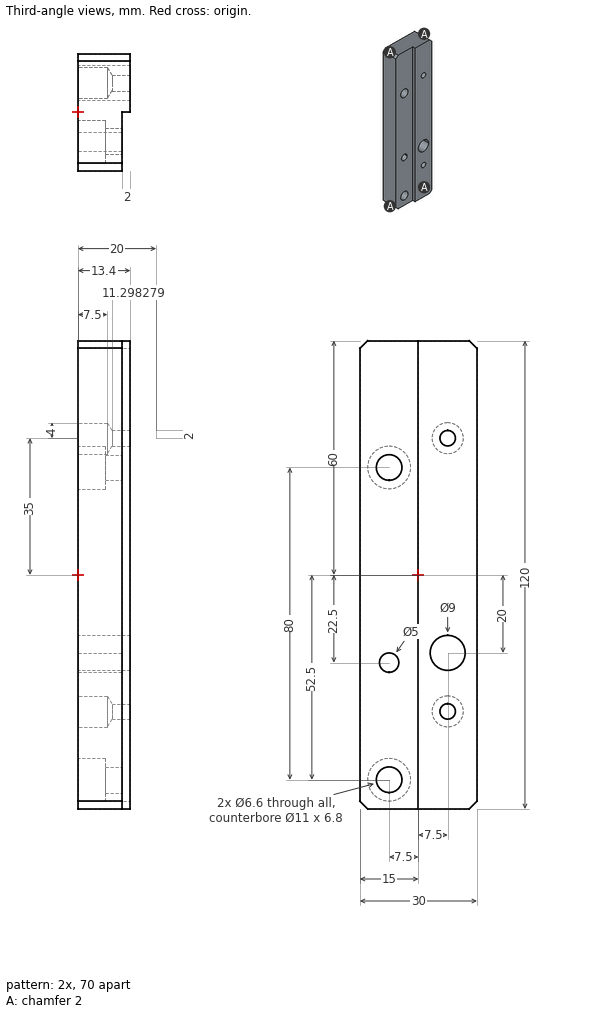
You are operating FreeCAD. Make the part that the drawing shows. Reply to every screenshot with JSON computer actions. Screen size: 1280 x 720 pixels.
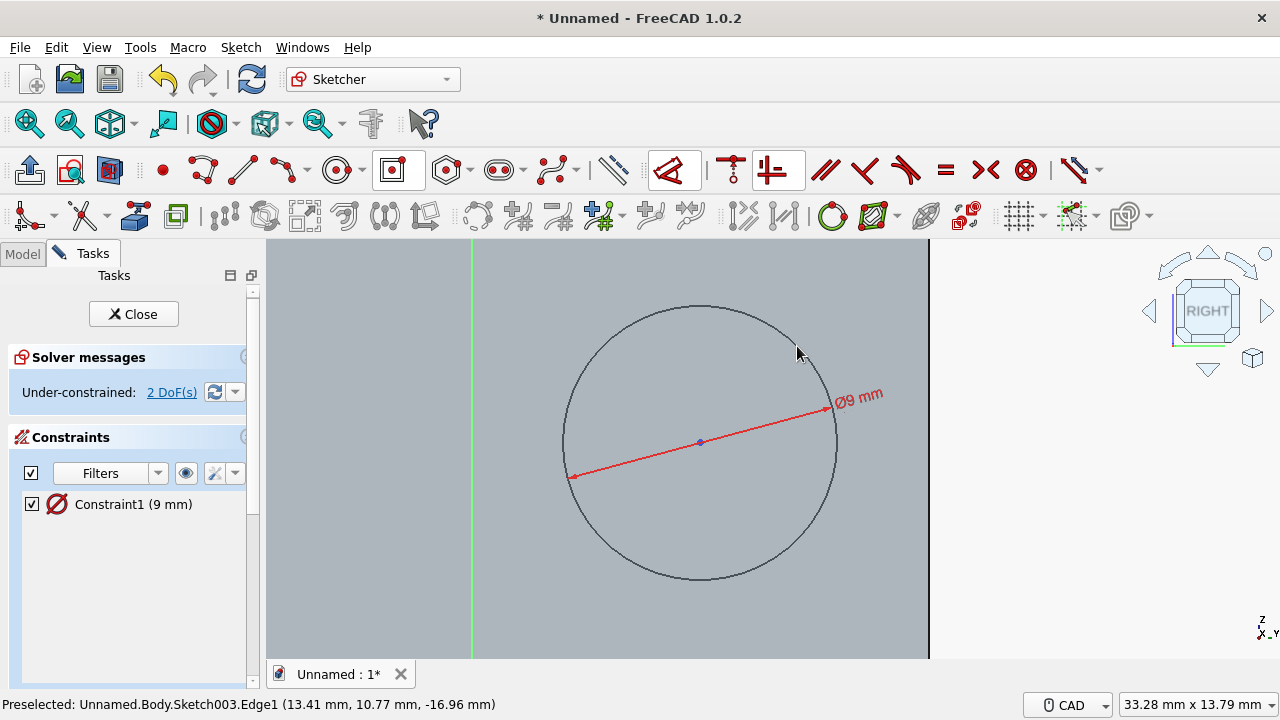
{"action": "left_click", "coordinate": [700, 443]}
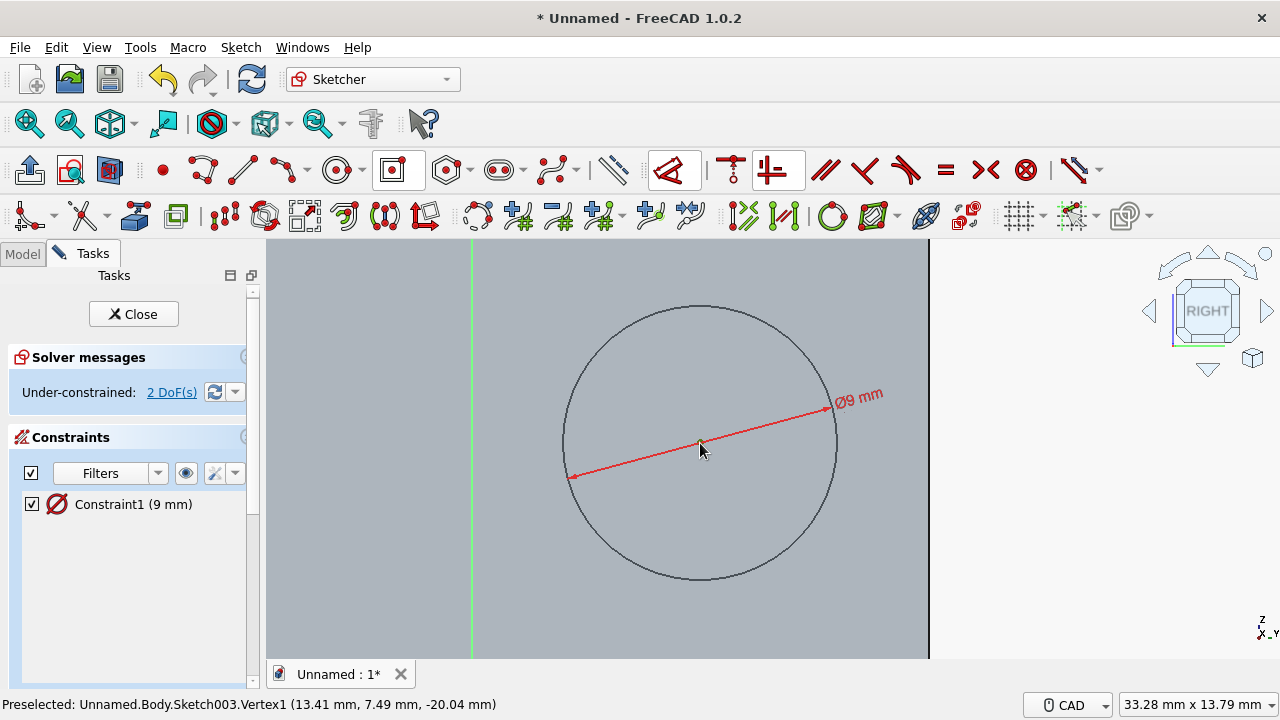
{"action": "left_click", "coordinate": [696, 170]}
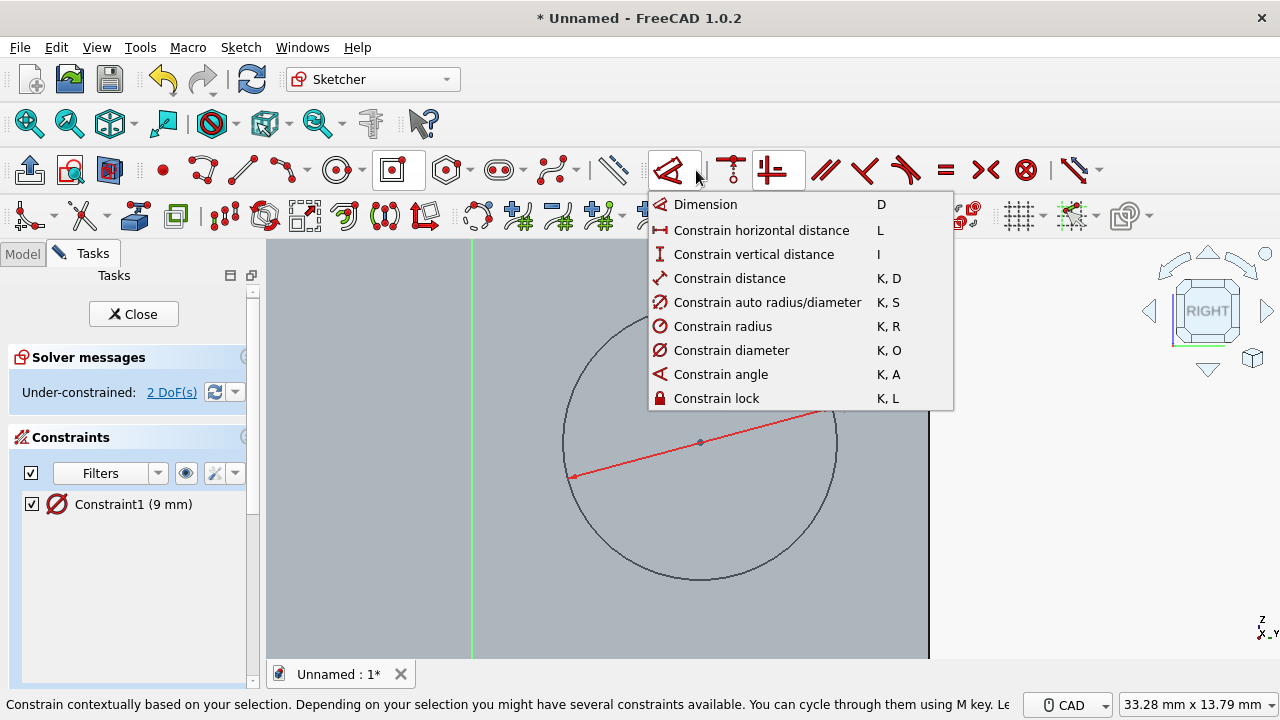
{"action": "left_click", "coordinate": [801, 254]}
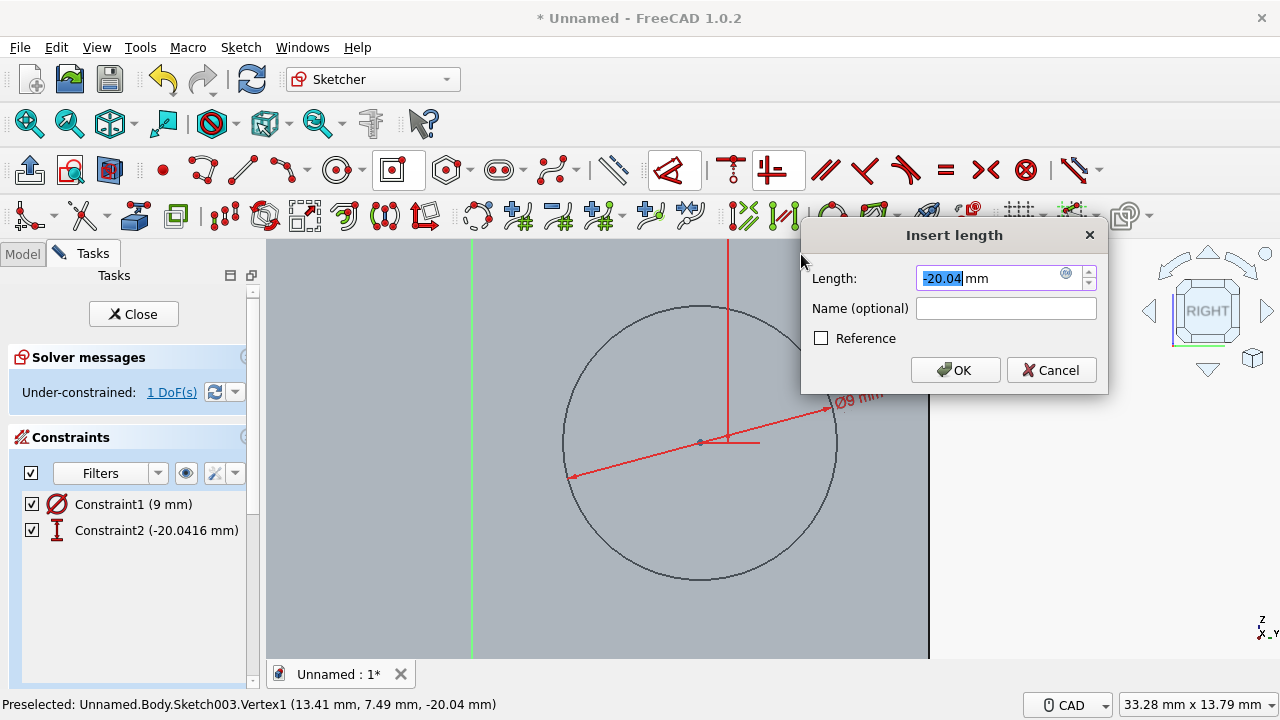
{"action": "type", "text": "-20"}
{"action": "key", "text": "Return"}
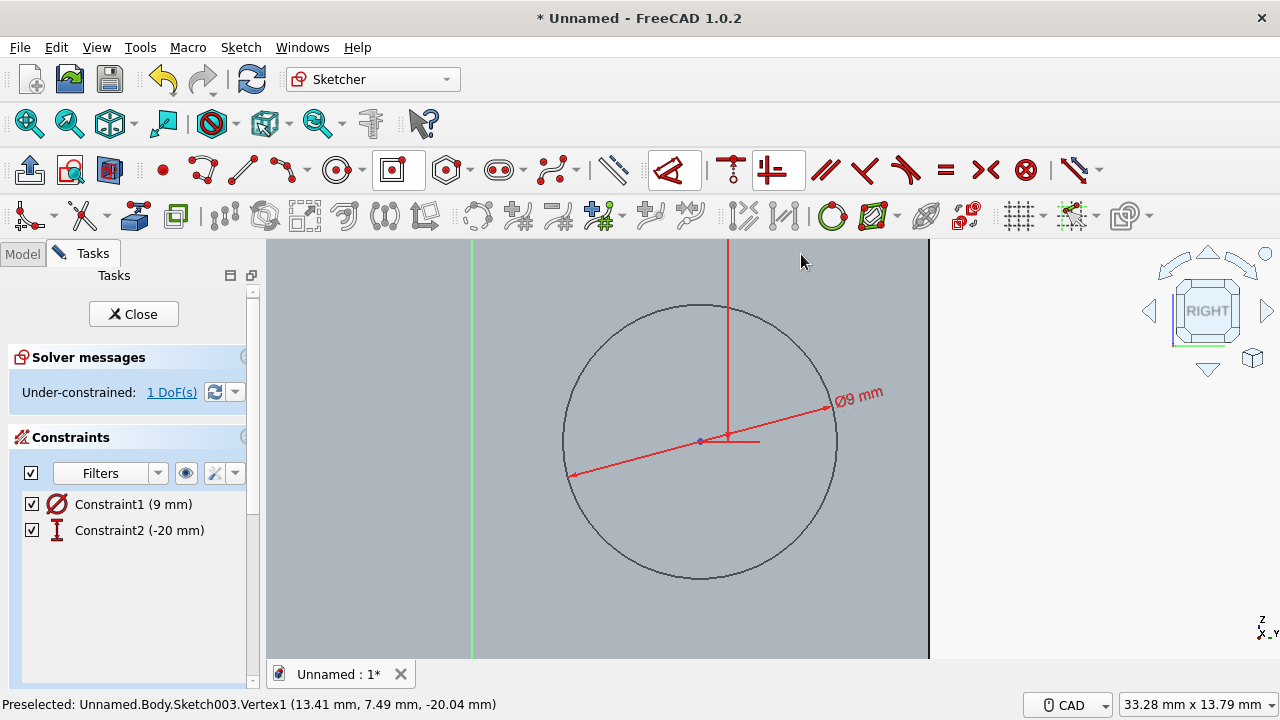
{"action": "left_click", "coordinate": [700, 442]}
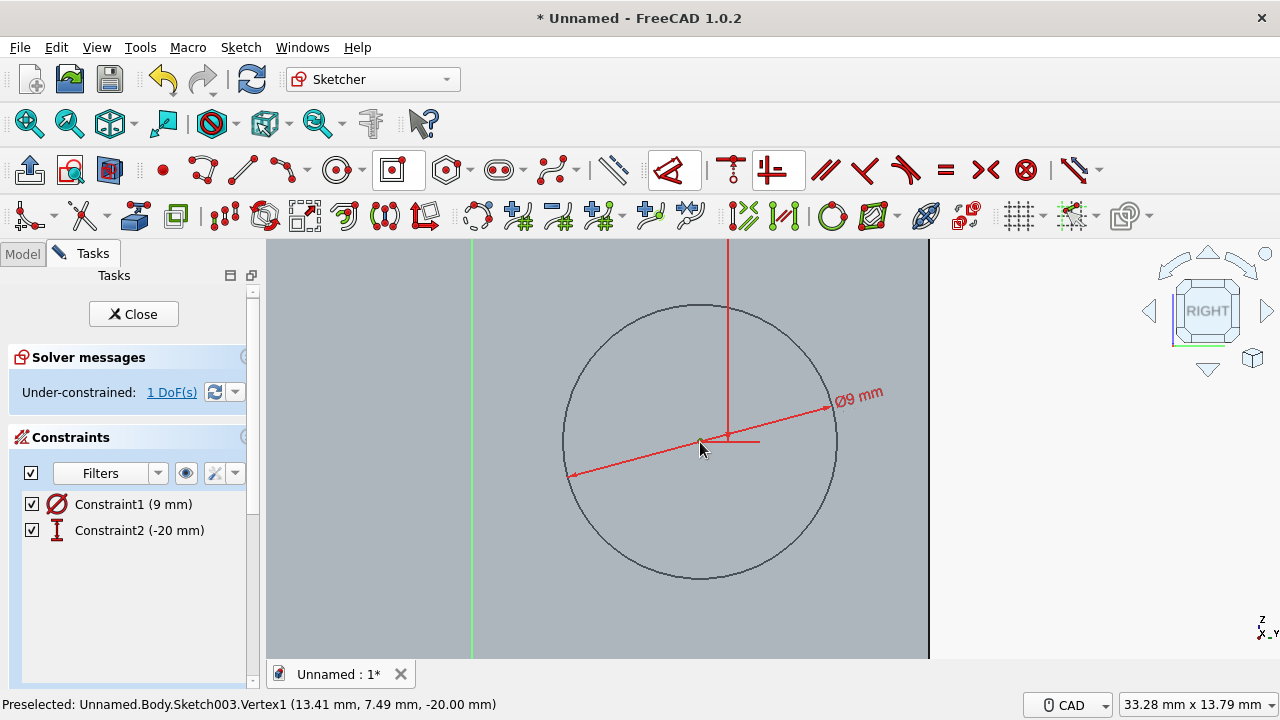
{"action": "key", "text": "l"}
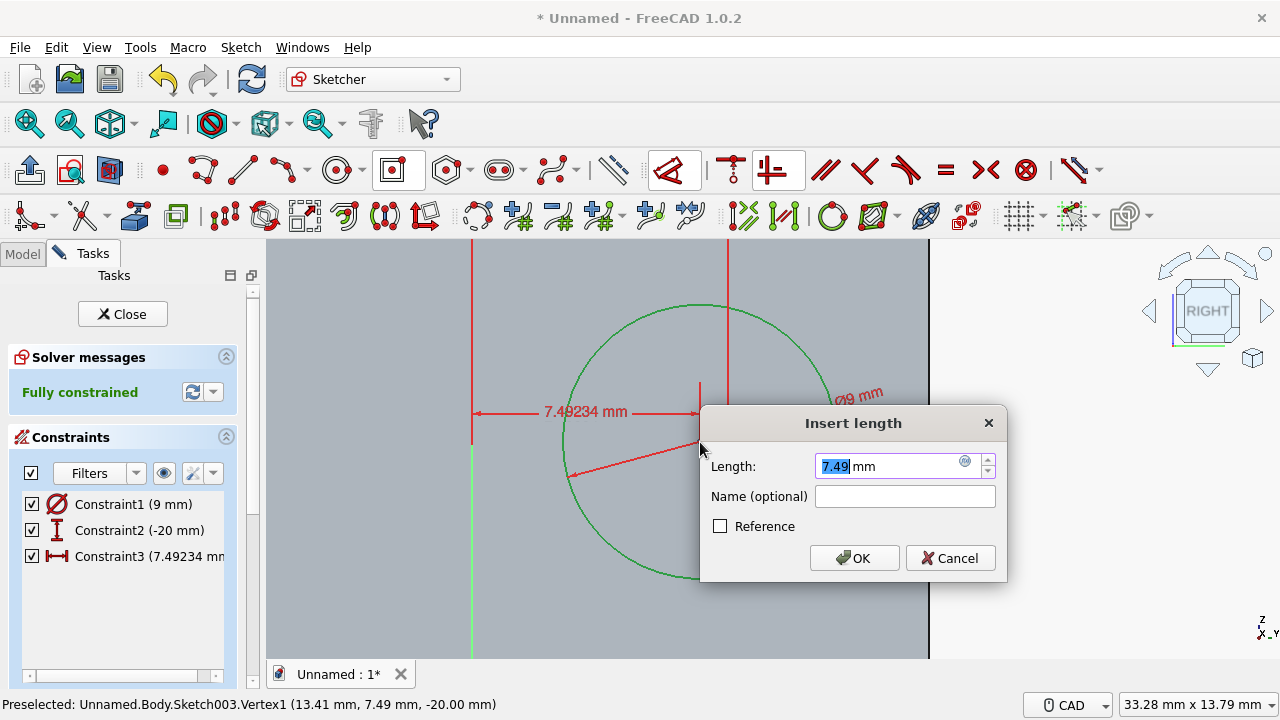
{"action": "type", "text": "7.5"}
{"action": "key", "text": "Return"}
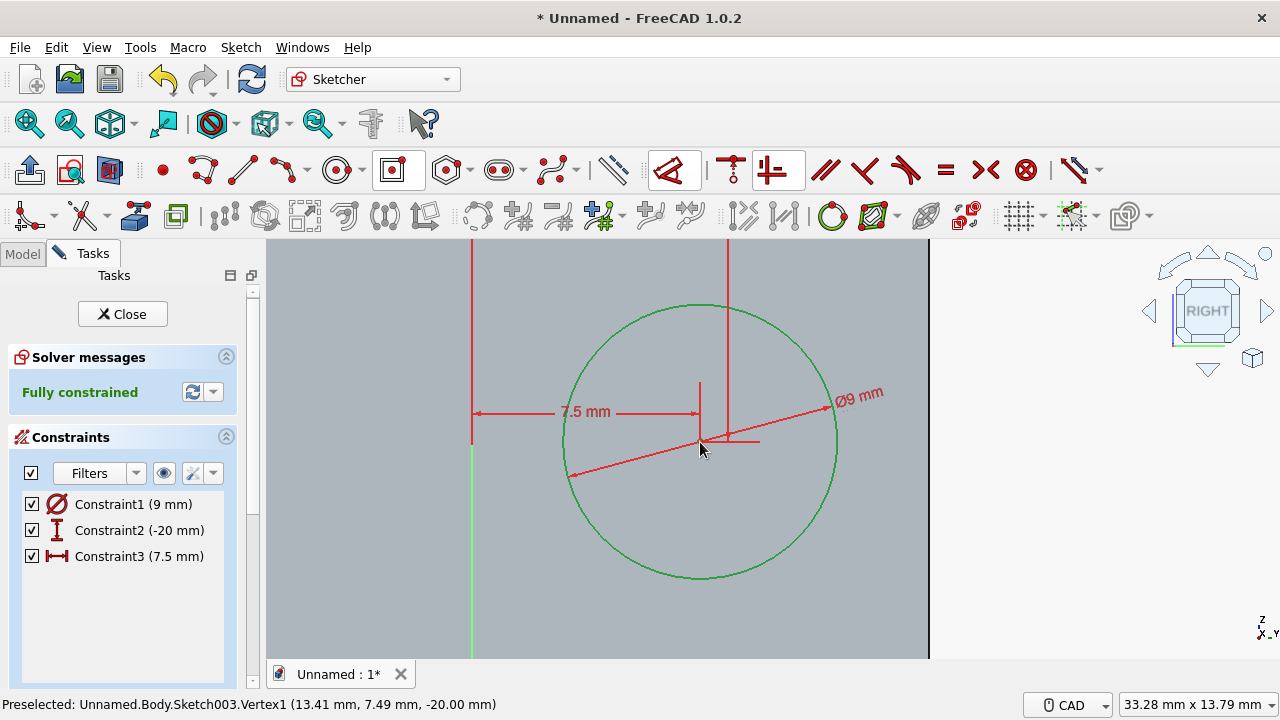
{"action": "left_click", "coordinate": [123, 314]}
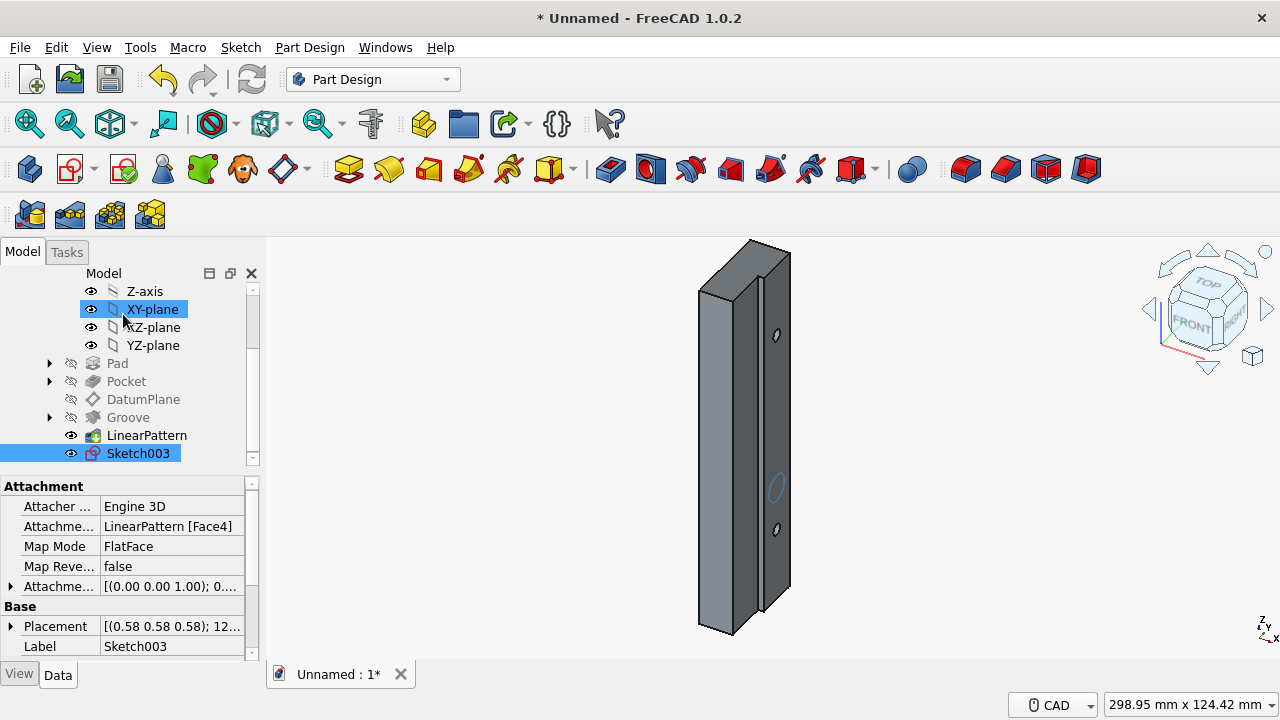
{"action": "left_click", "coordinate": [612, 170]}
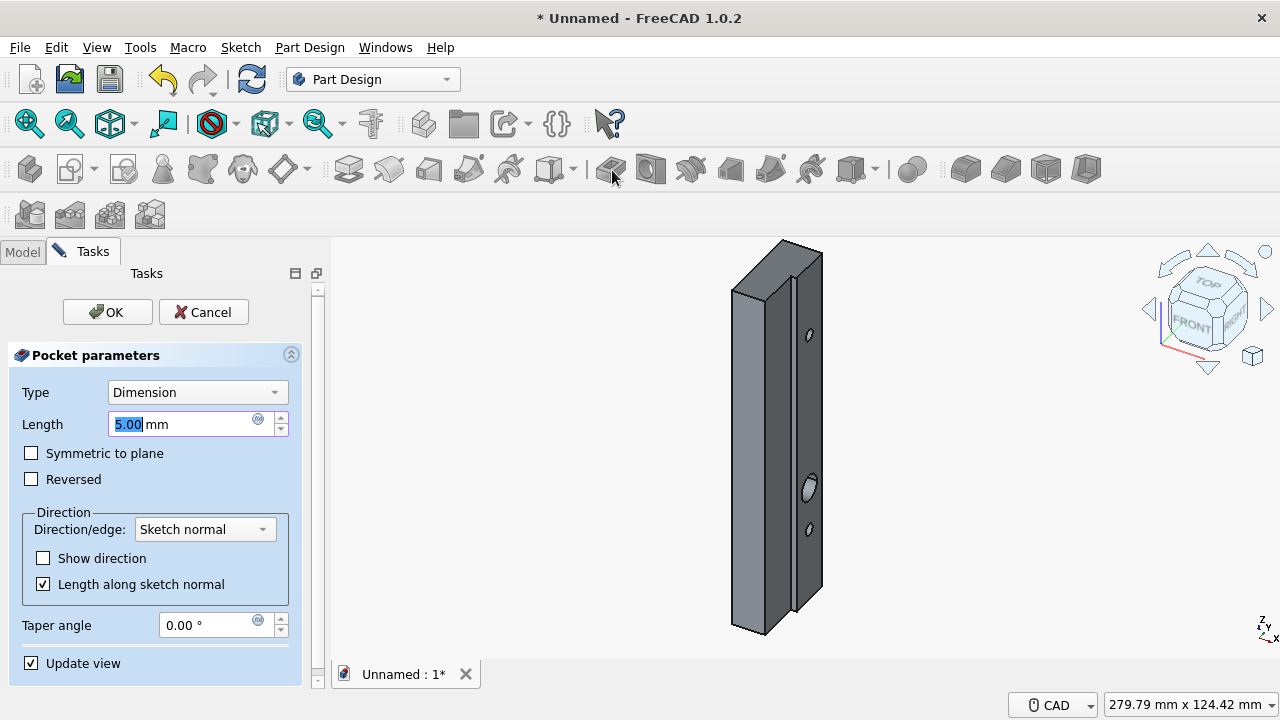
{"action": "left_click", "coordinate": [198, 392]}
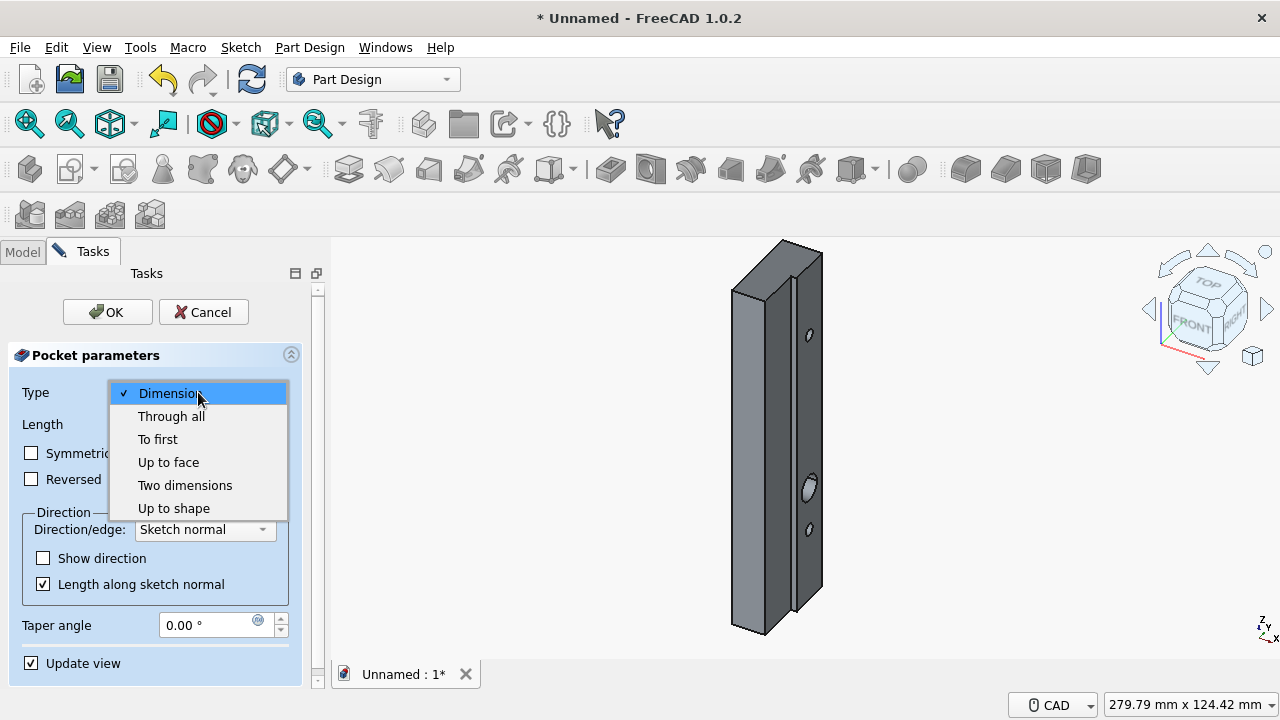
{"action": "left_click", "coordinate": [198, 416]}